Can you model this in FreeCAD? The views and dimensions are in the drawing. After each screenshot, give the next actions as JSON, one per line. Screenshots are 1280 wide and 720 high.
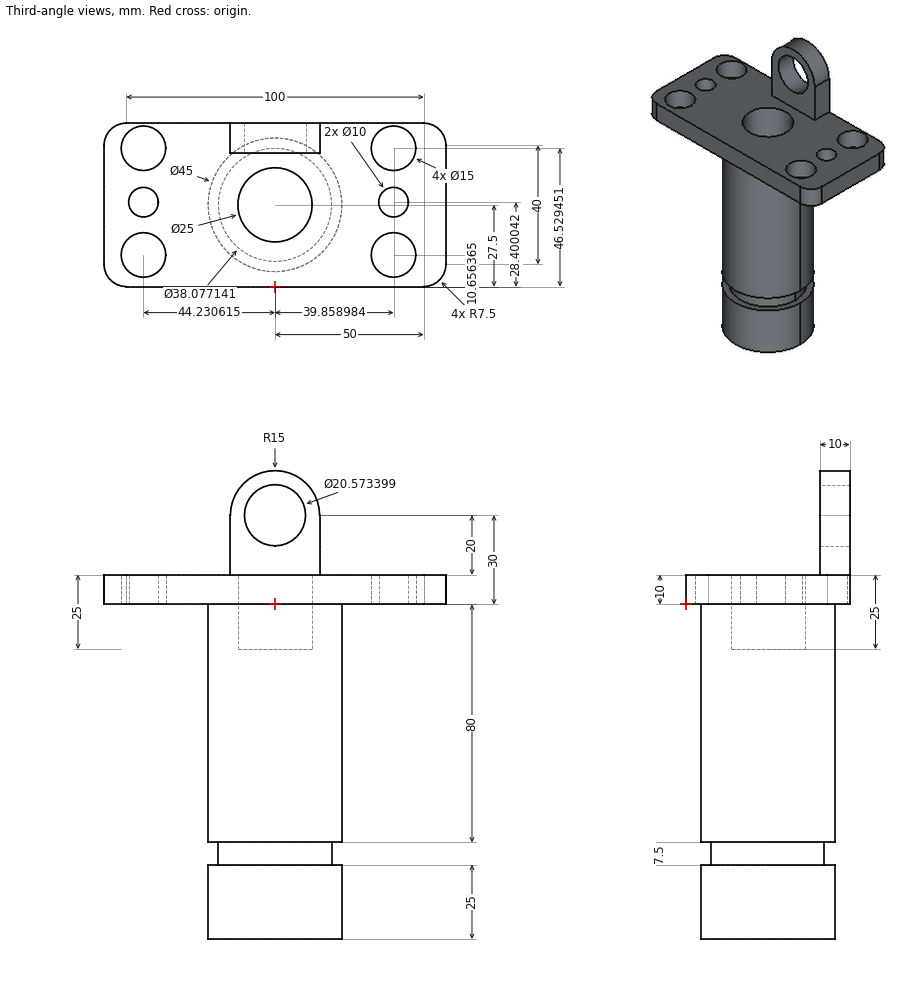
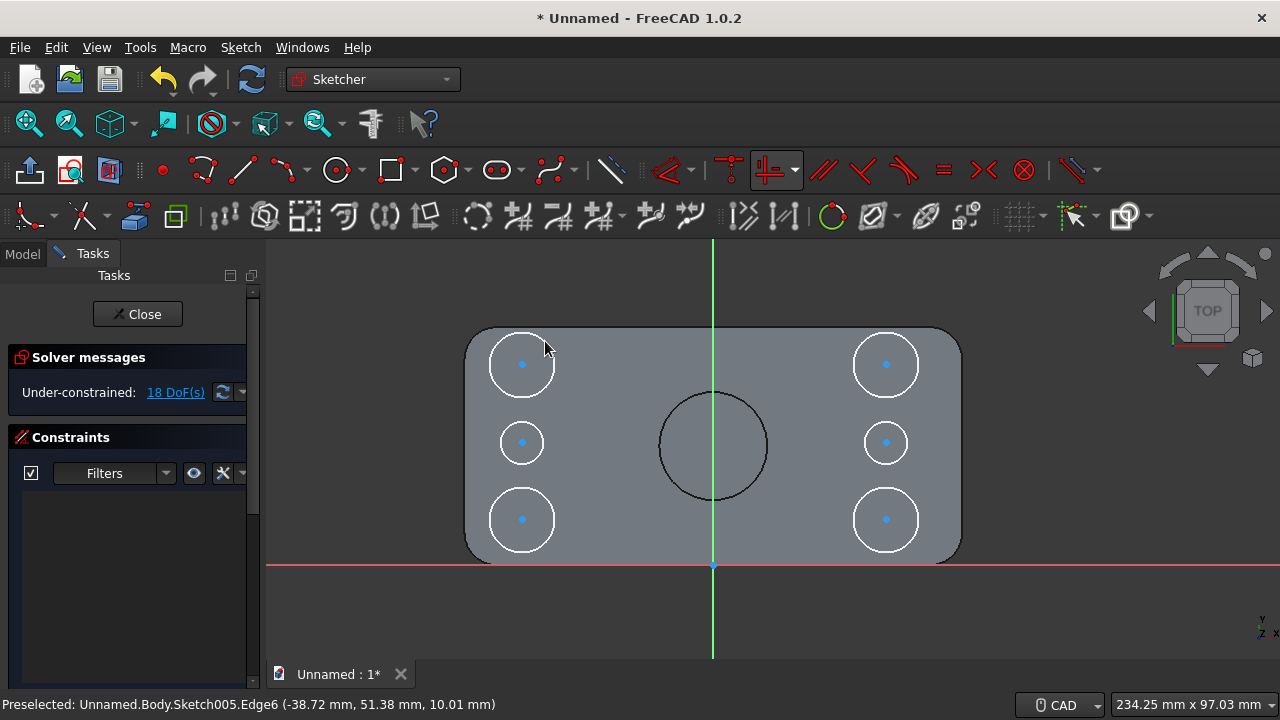
{"action": "left_click", "coordinate": [909, 342]}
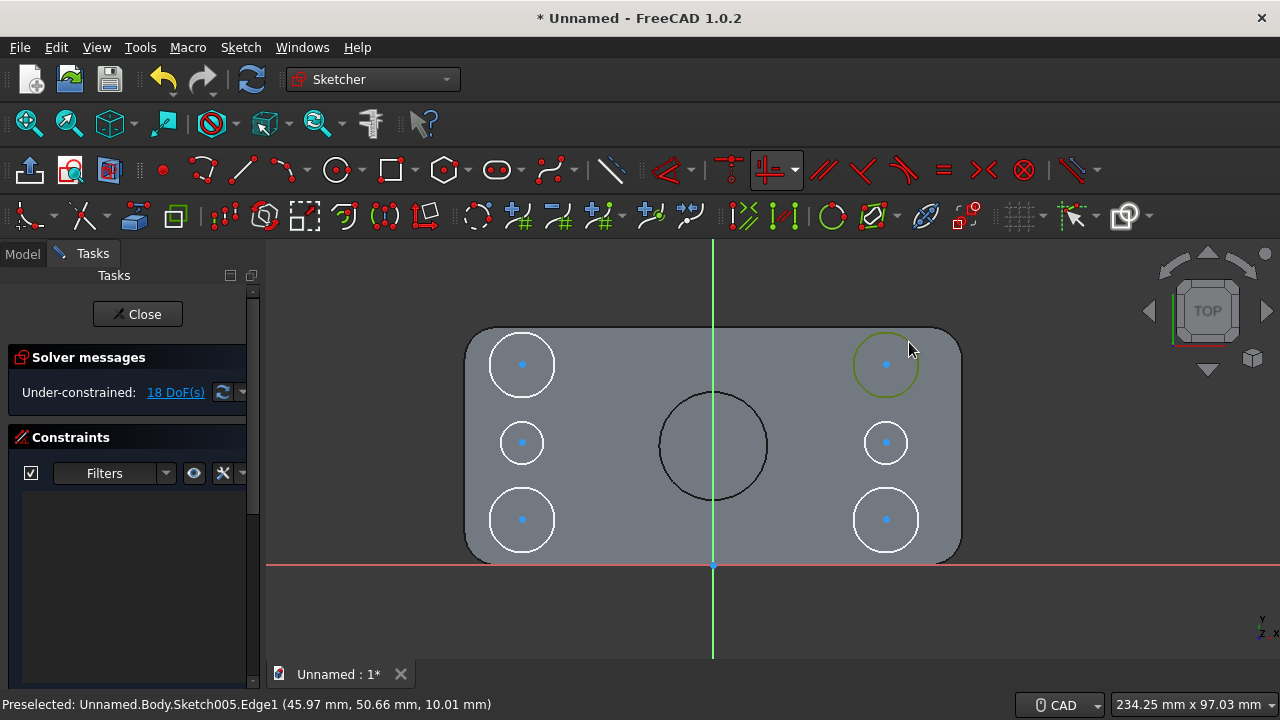
{"action": "left_click", "coordinate": [909, 497]}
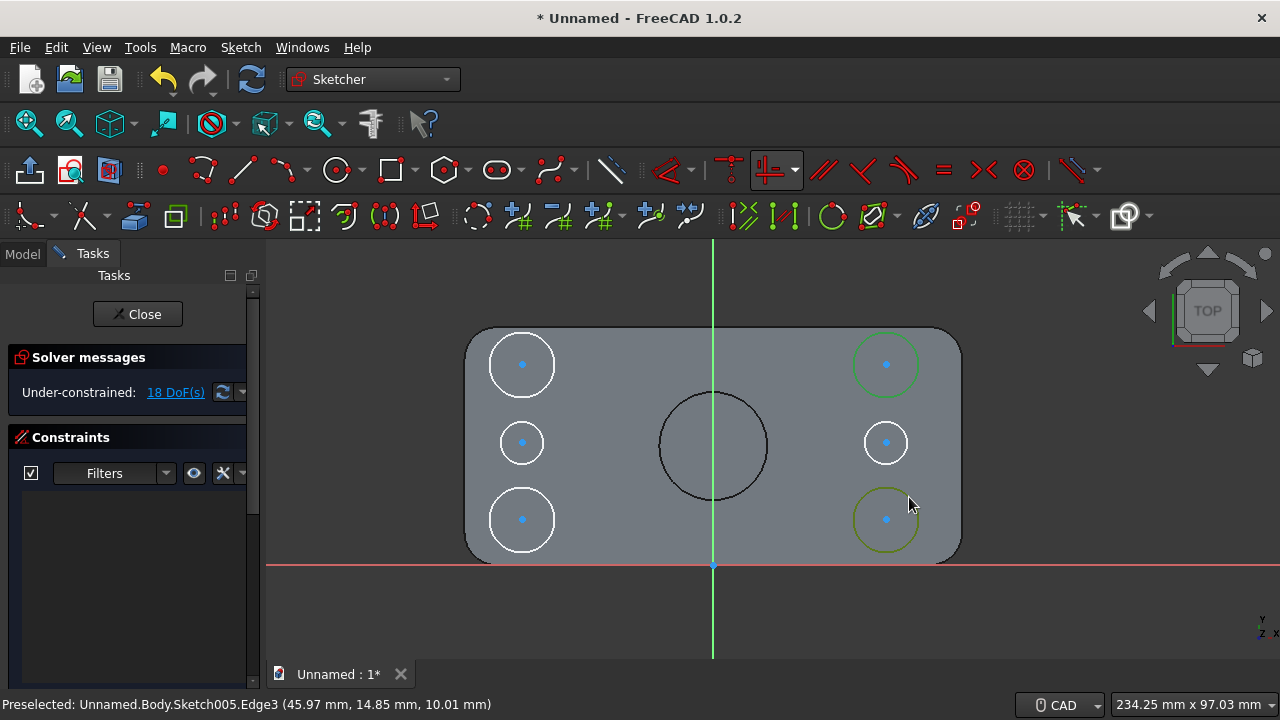
{"action": "left_click", "coordinate": [545, 497]}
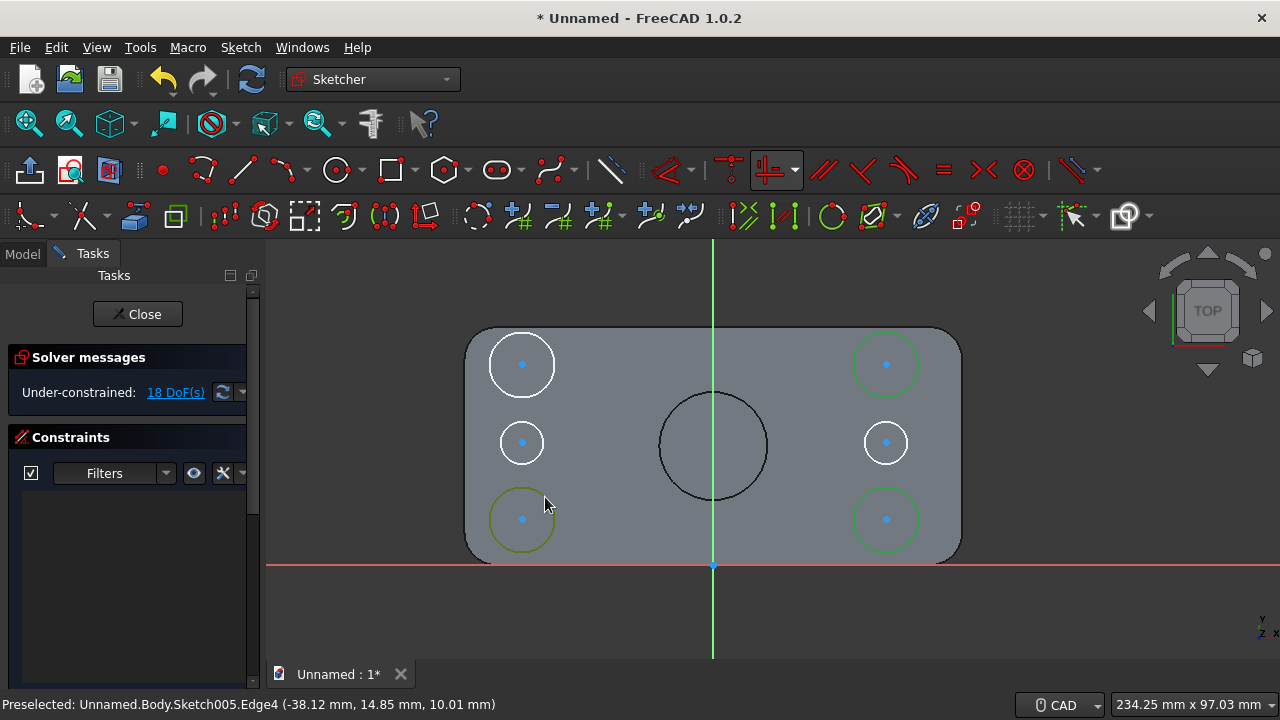
{"action": "left_click", "coordinate": [545, 342]}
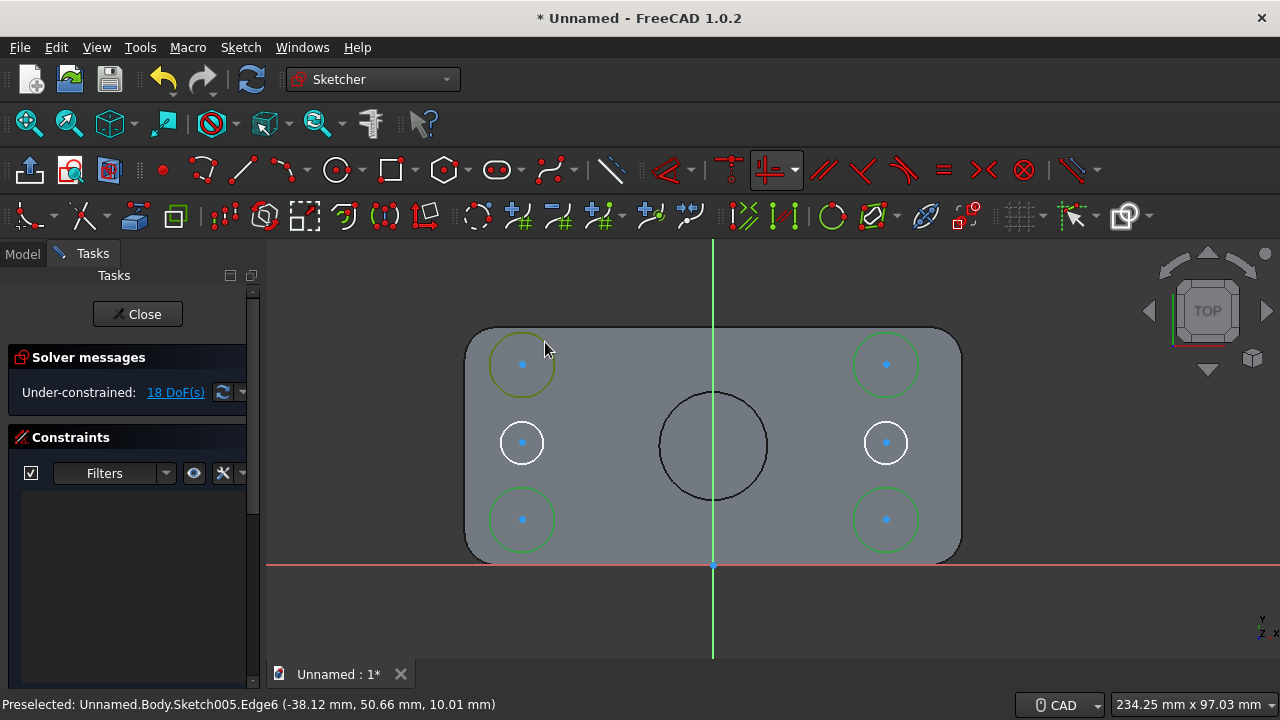
{"action": "left_click", "coordinate": [944, 170]}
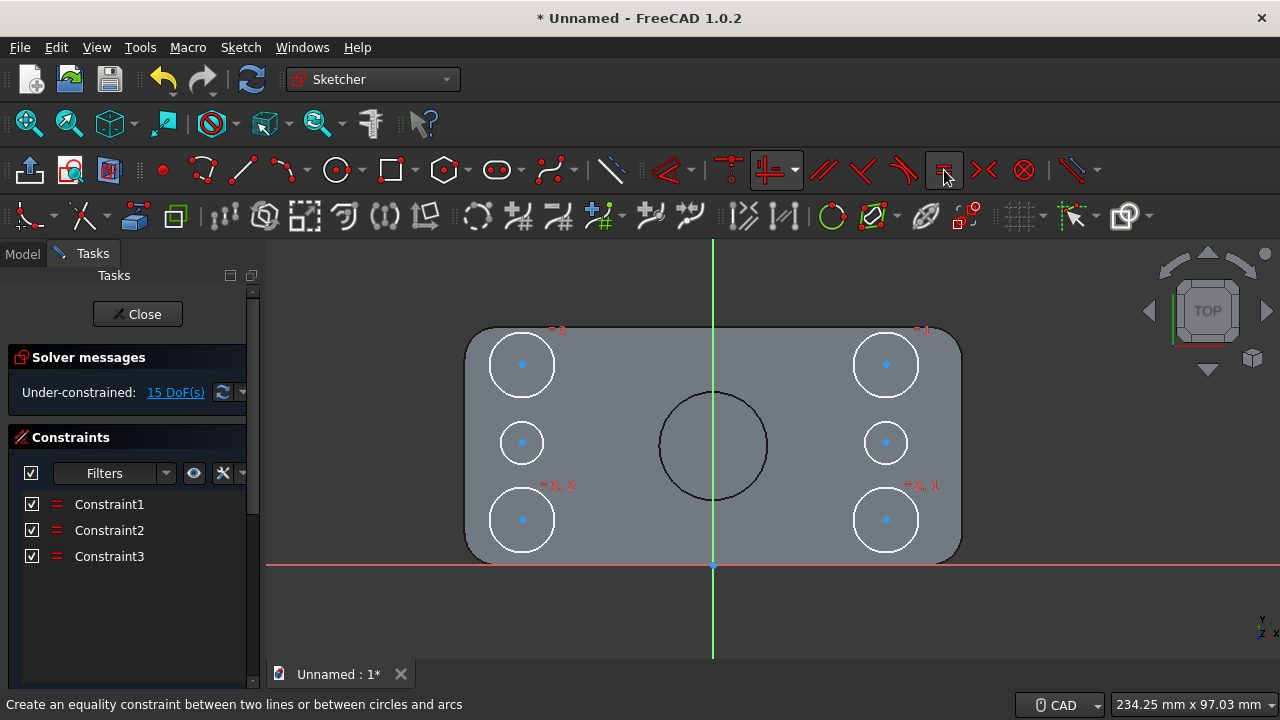
{"action": "left_click", "coordinate": [901, 428]}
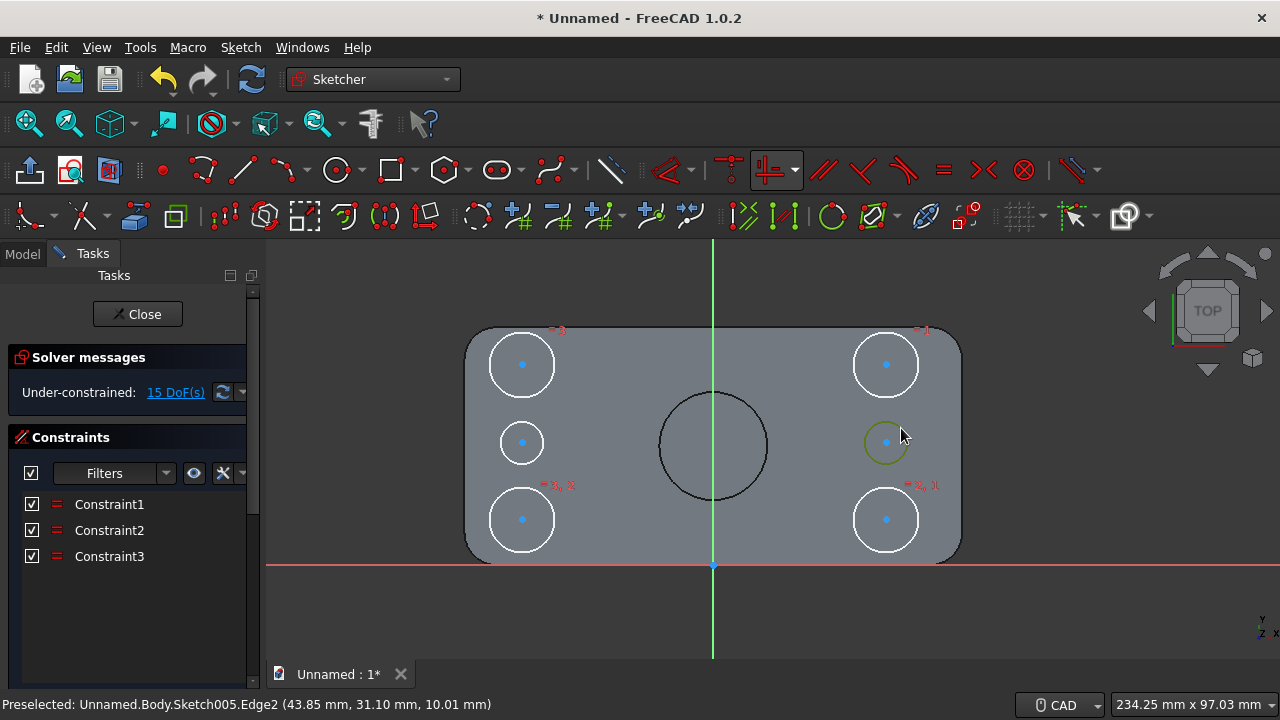
{"action": "left_click", "coordinate": [537, 428]}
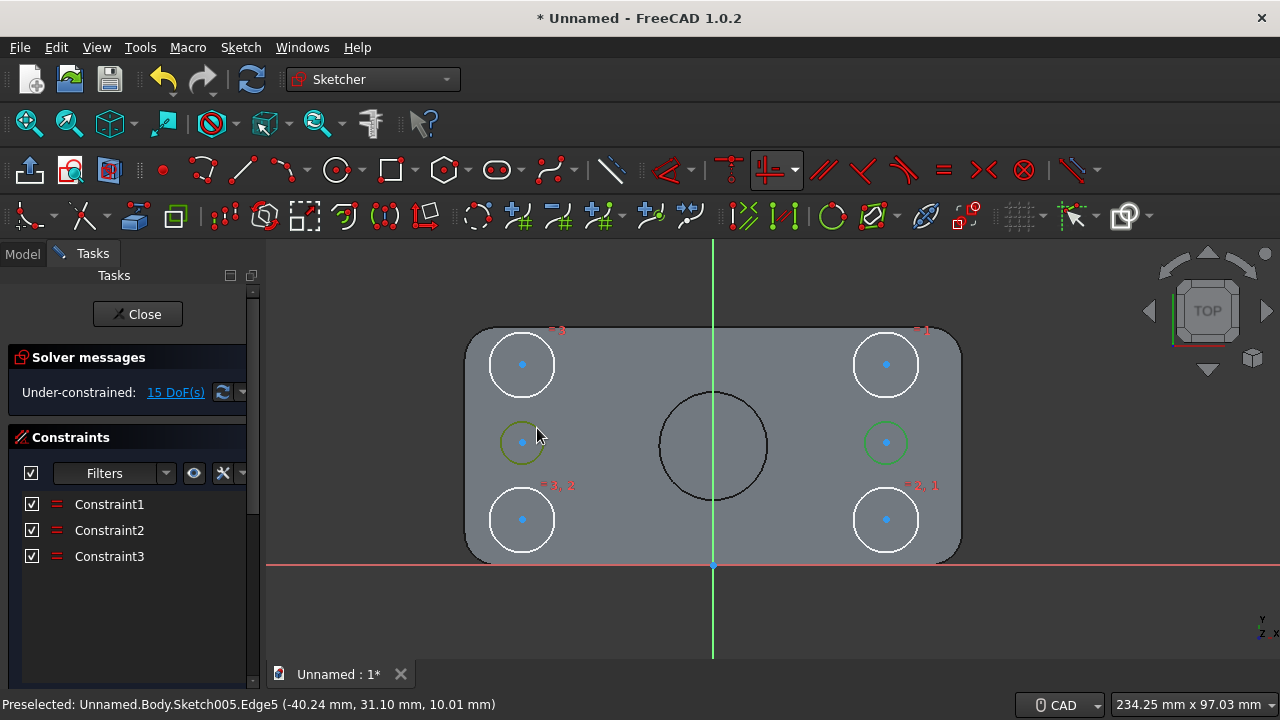
{"action": "key", "text": "e"}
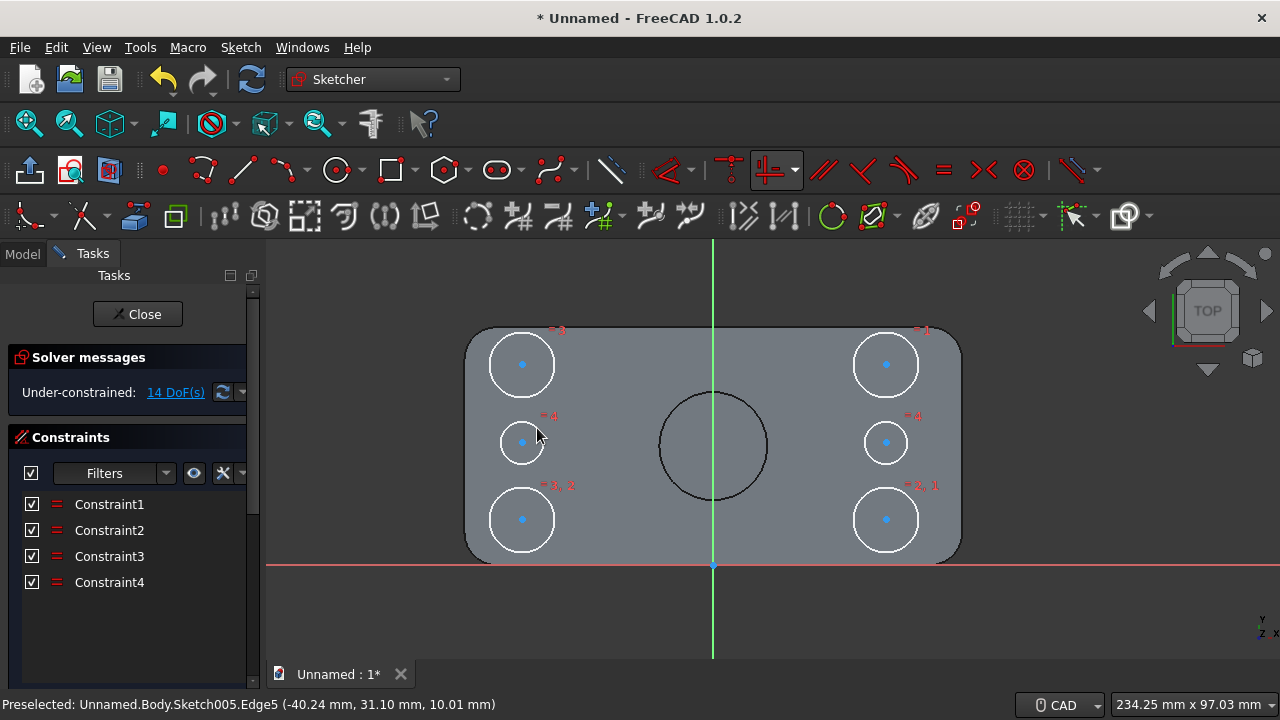
{"action": "left_click", "coordinate": [886, 365]}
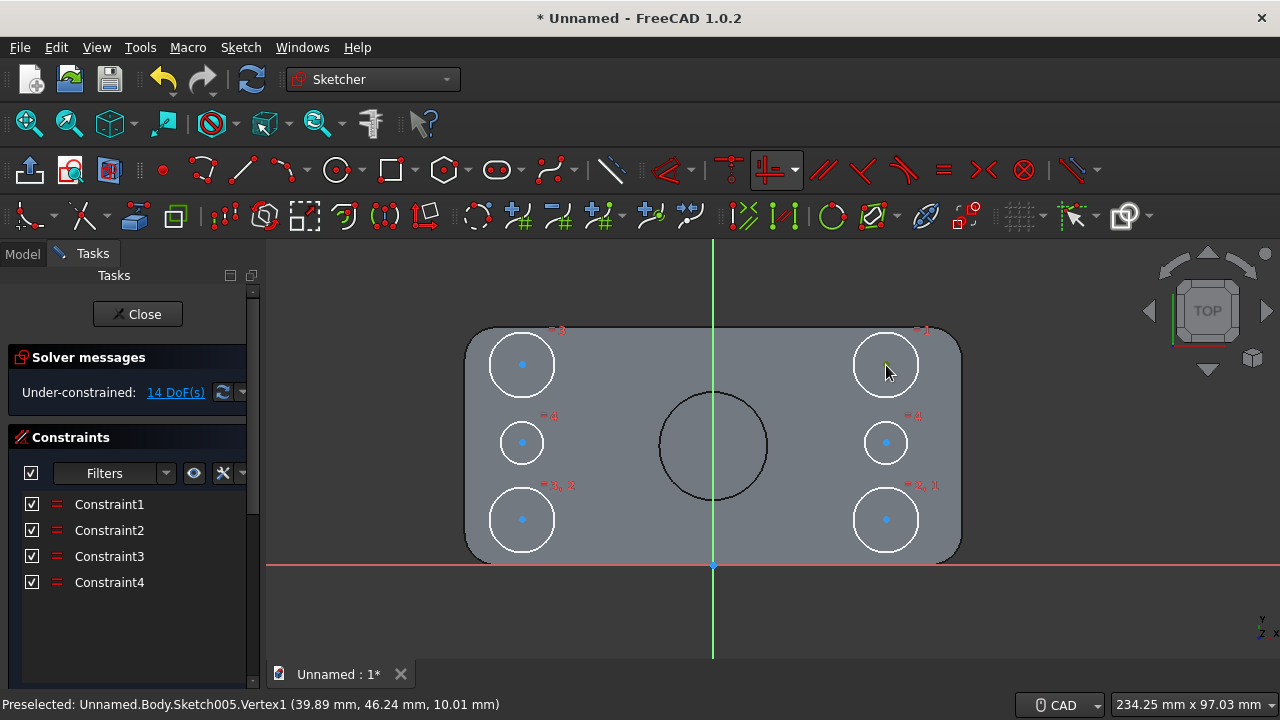
{"action": "left_click", "coordinate": [886, 443]}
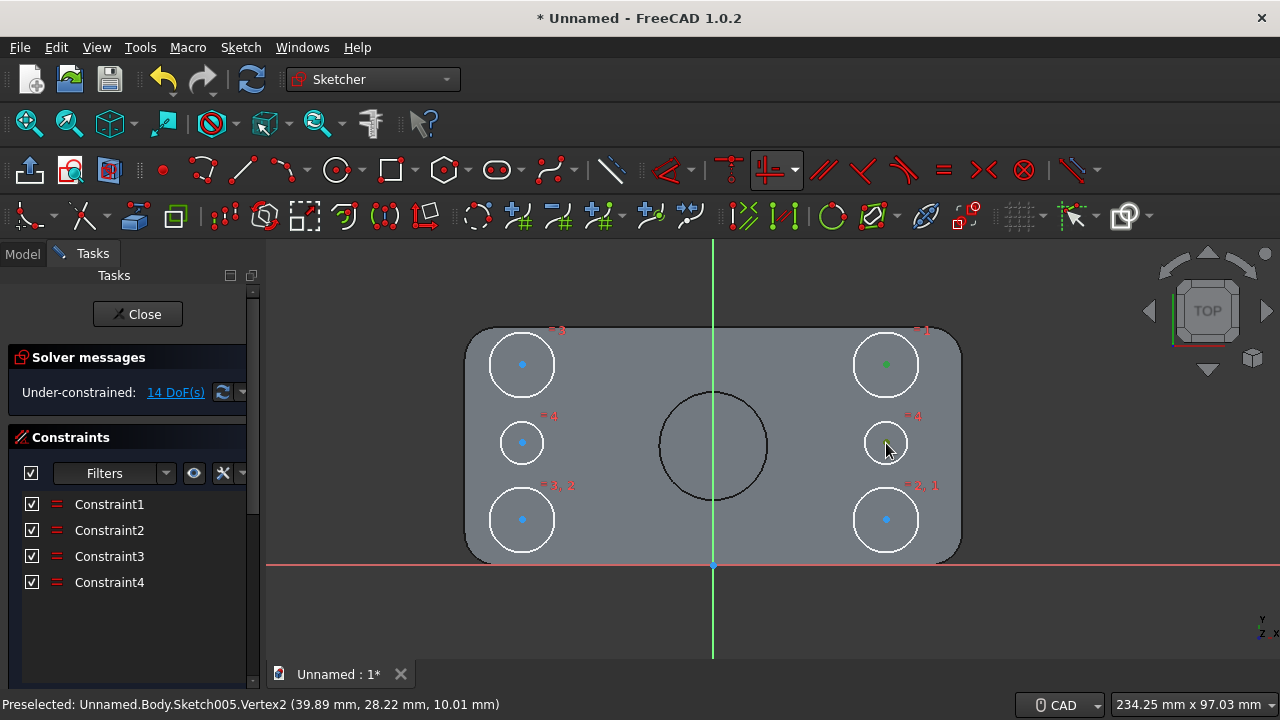
{"action": "key", "text": "v"}